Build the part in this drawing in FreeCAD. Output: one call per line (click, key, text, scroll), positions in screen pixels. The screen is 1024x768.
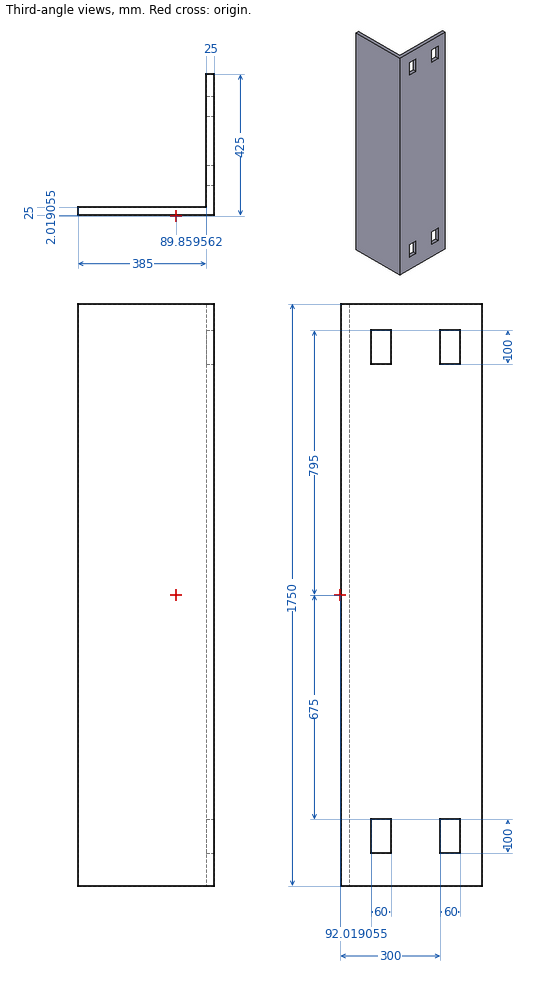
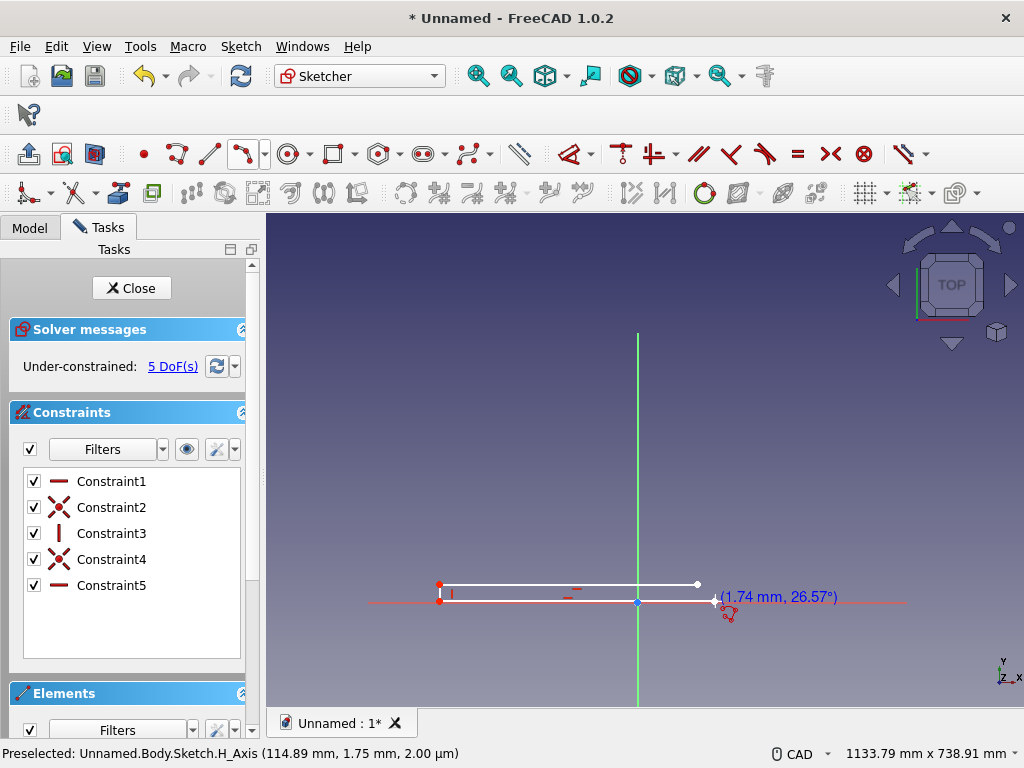
click(715, 318)
click(698, 318)
click(698, 585)
key(Escape)
key(Escape)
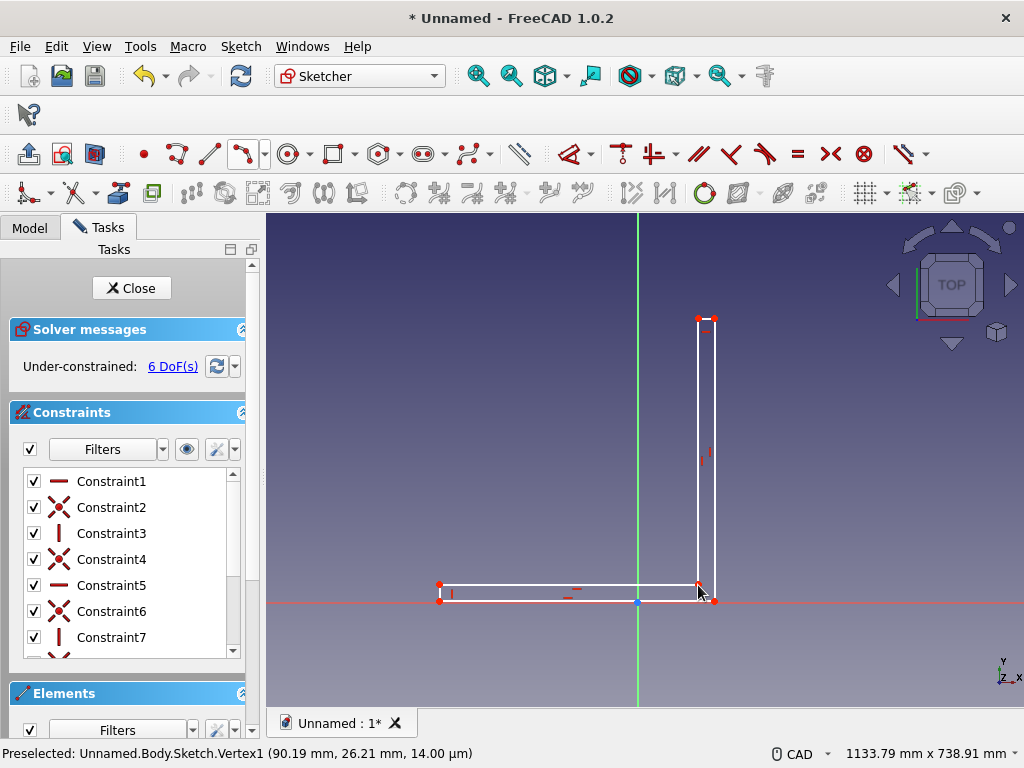
click(568, 154)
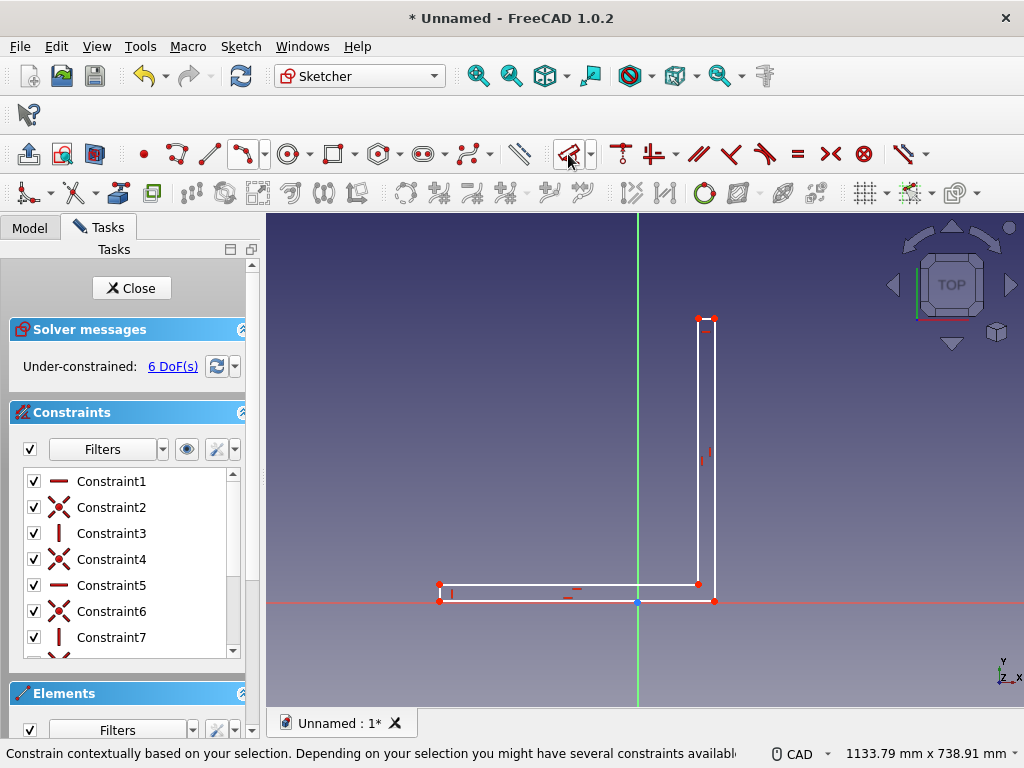
scroll(440, 593, up, 5)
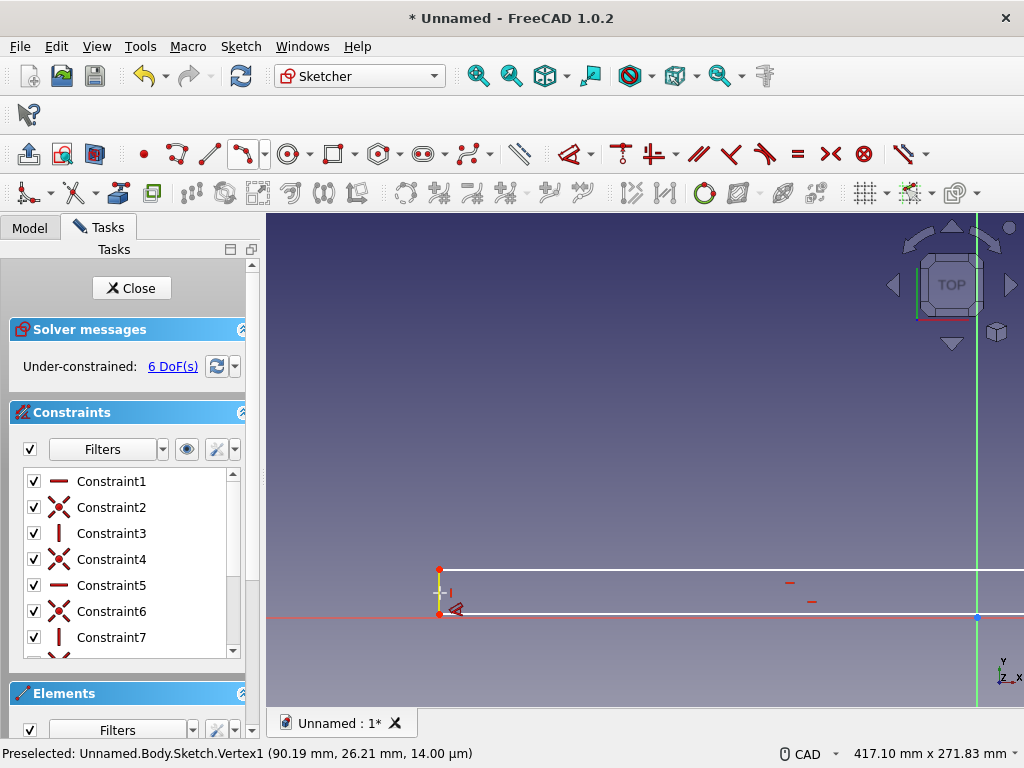
click(439, 592)
click(405, 592)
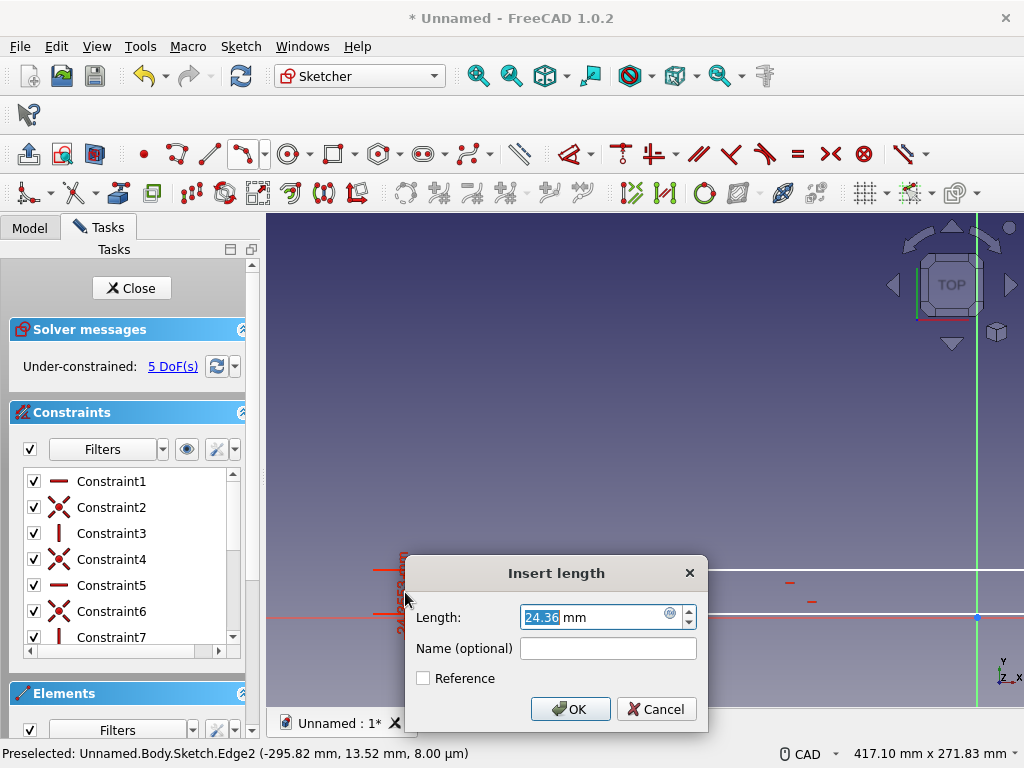
text(25)
key(Return)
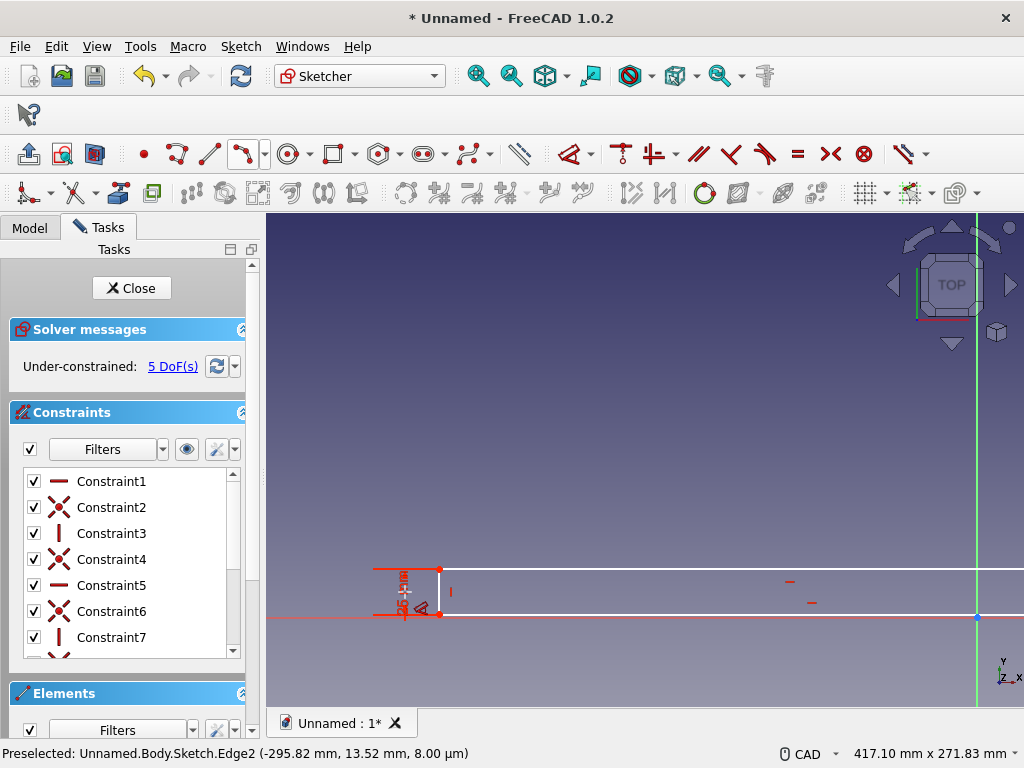
scroll(439, 593, down, 5)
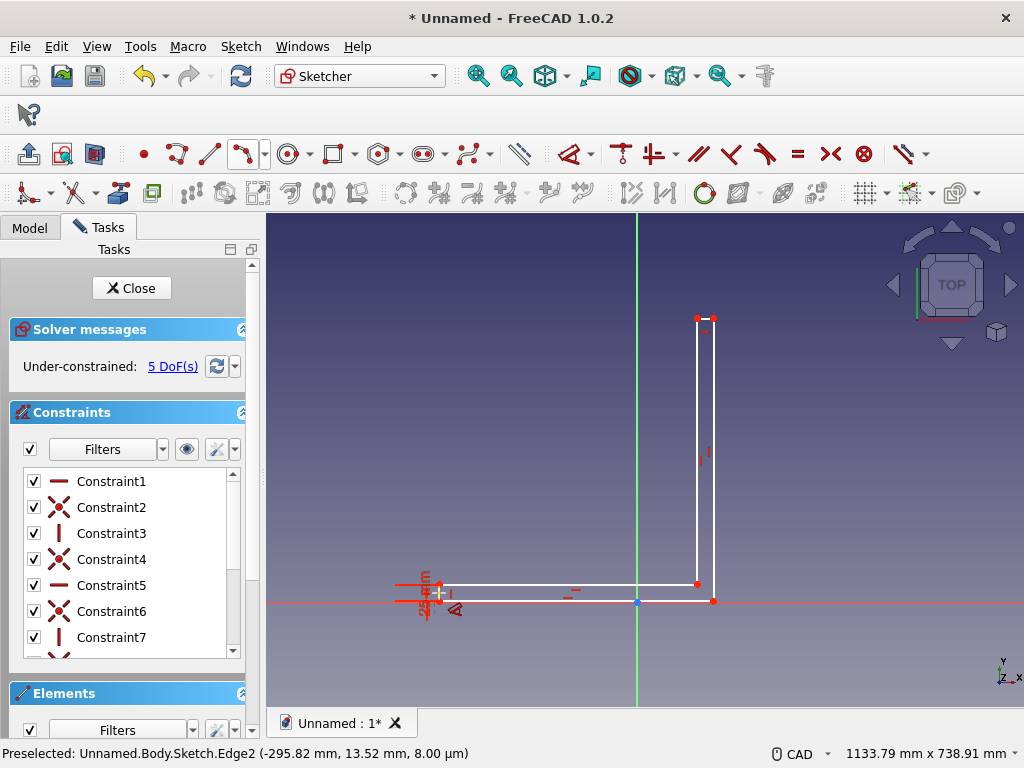
scroll(709, 319, up, 6)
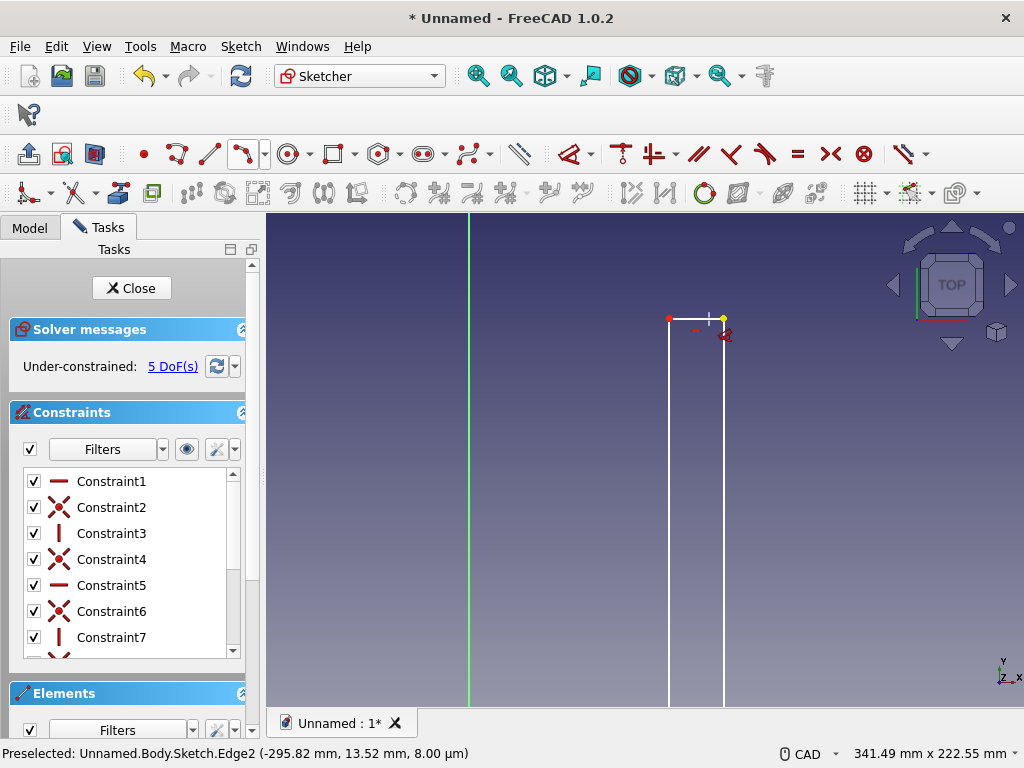
click(707, 319)
click(696, 285)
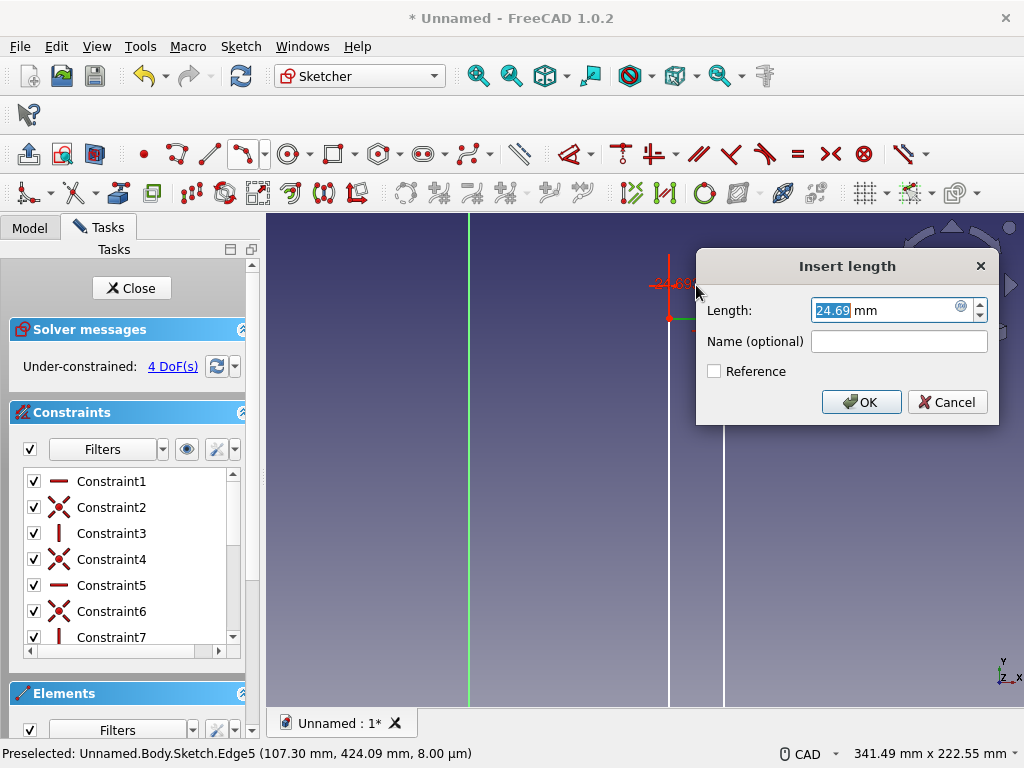
text(25)
key(Return)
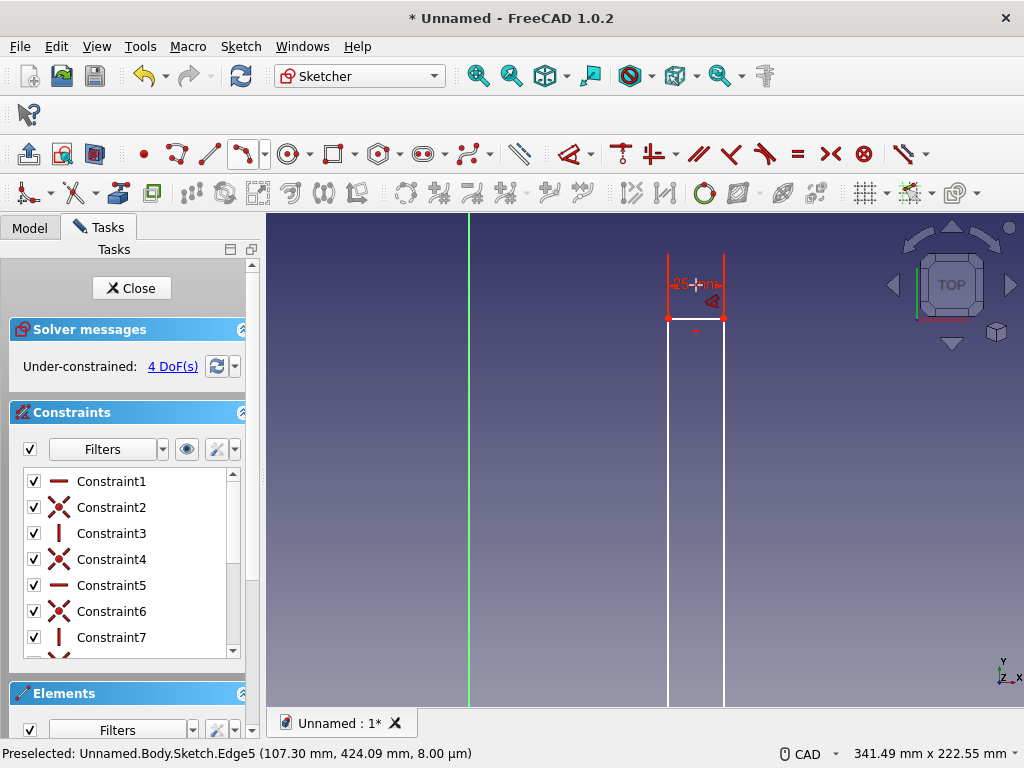
scroll(709, 319, down, 6)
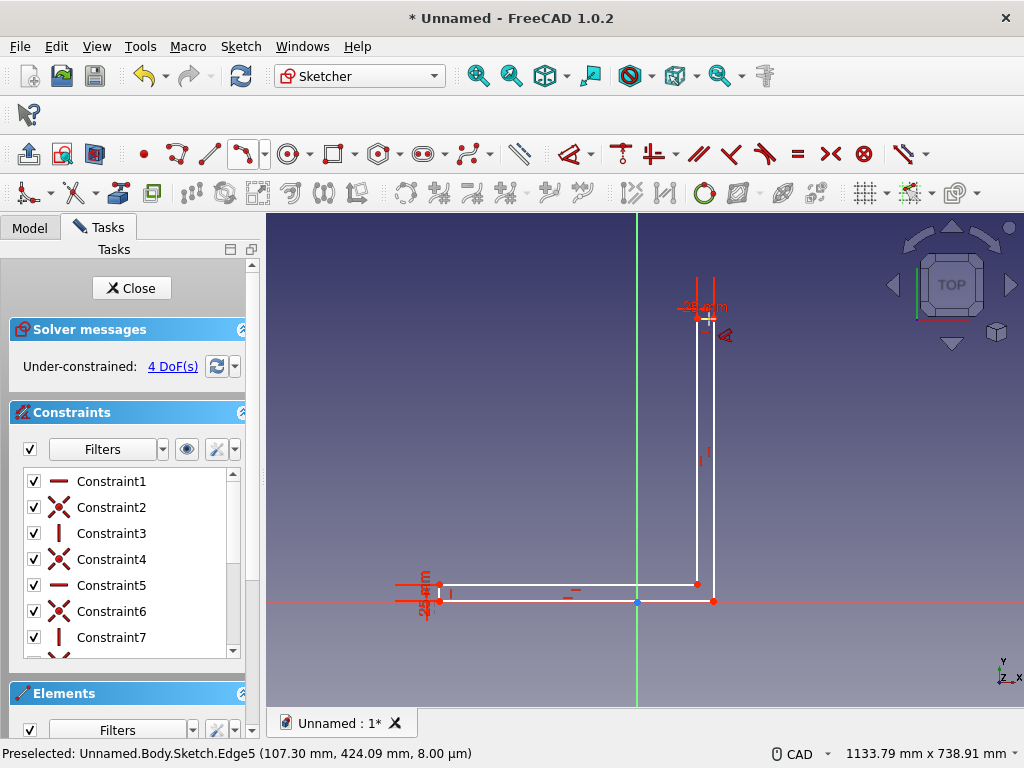
click(620, 585)
click(568, 619)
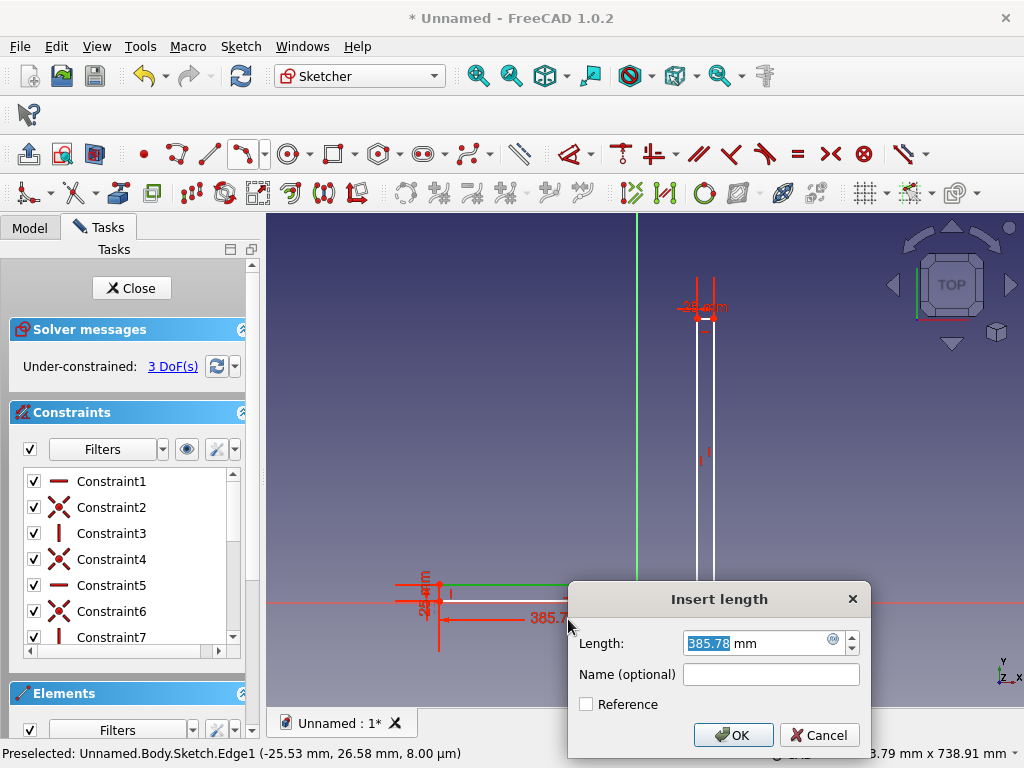
text(385)
key(Return)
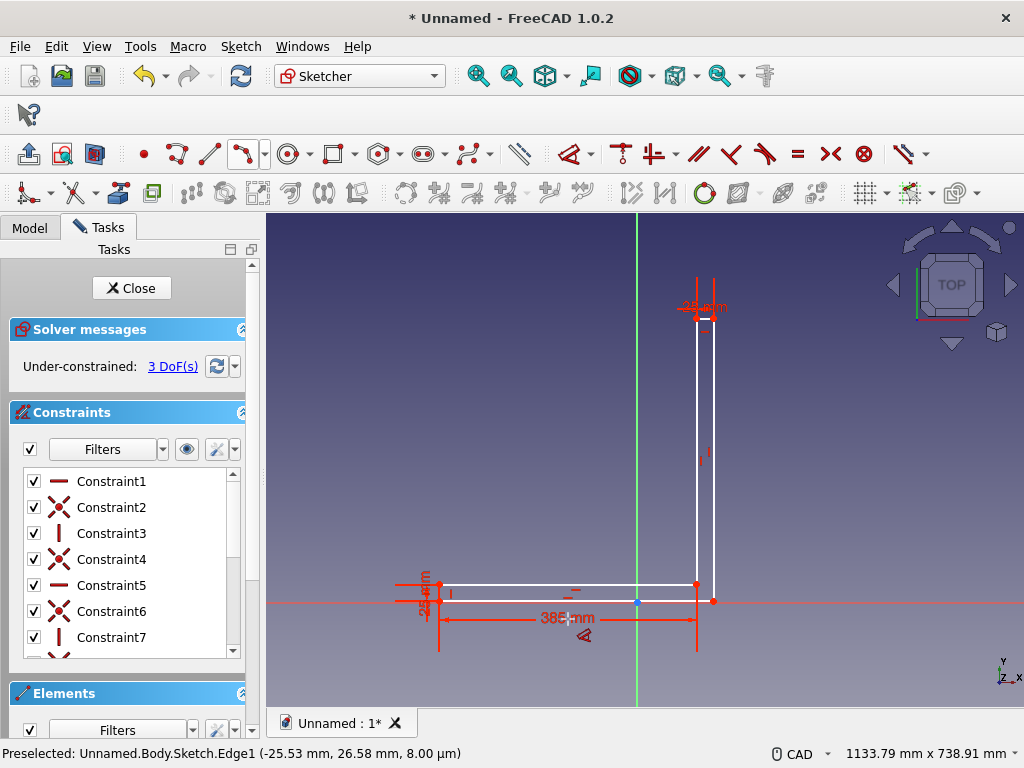
click(714, 319)
click(748, 461)